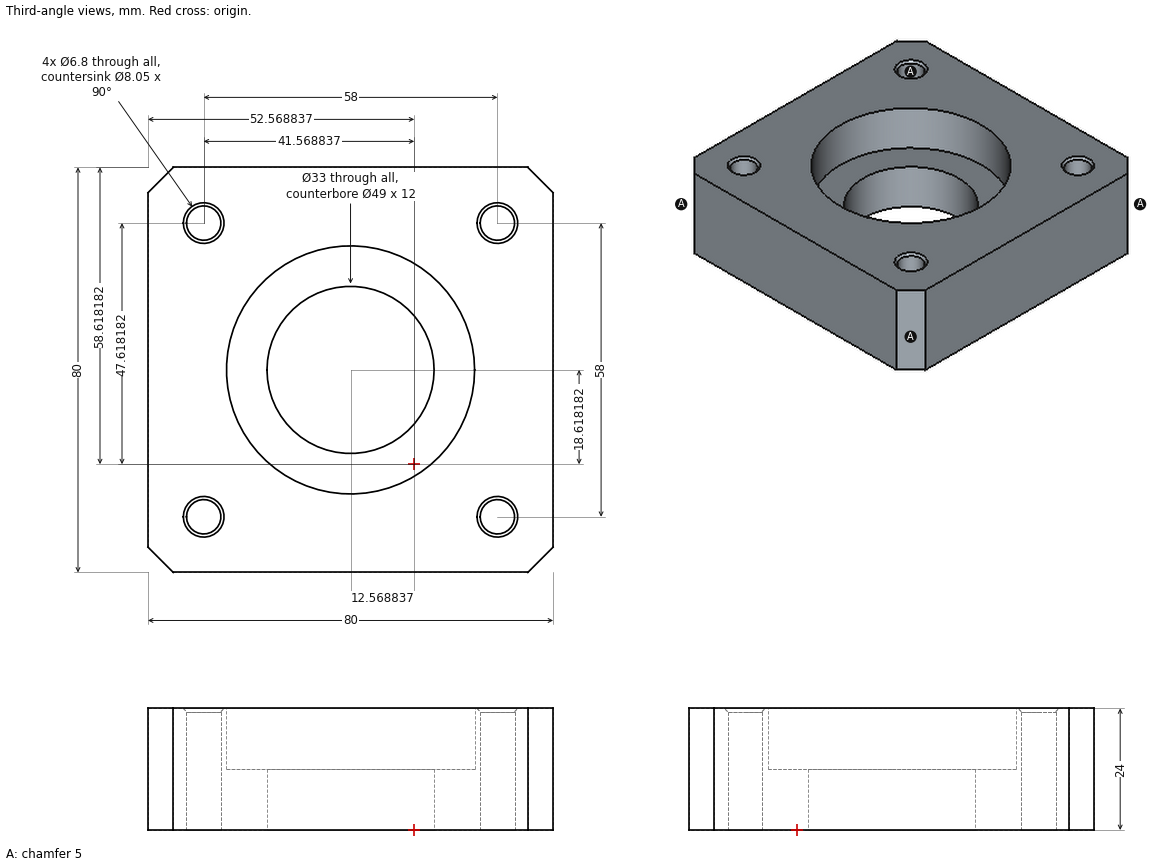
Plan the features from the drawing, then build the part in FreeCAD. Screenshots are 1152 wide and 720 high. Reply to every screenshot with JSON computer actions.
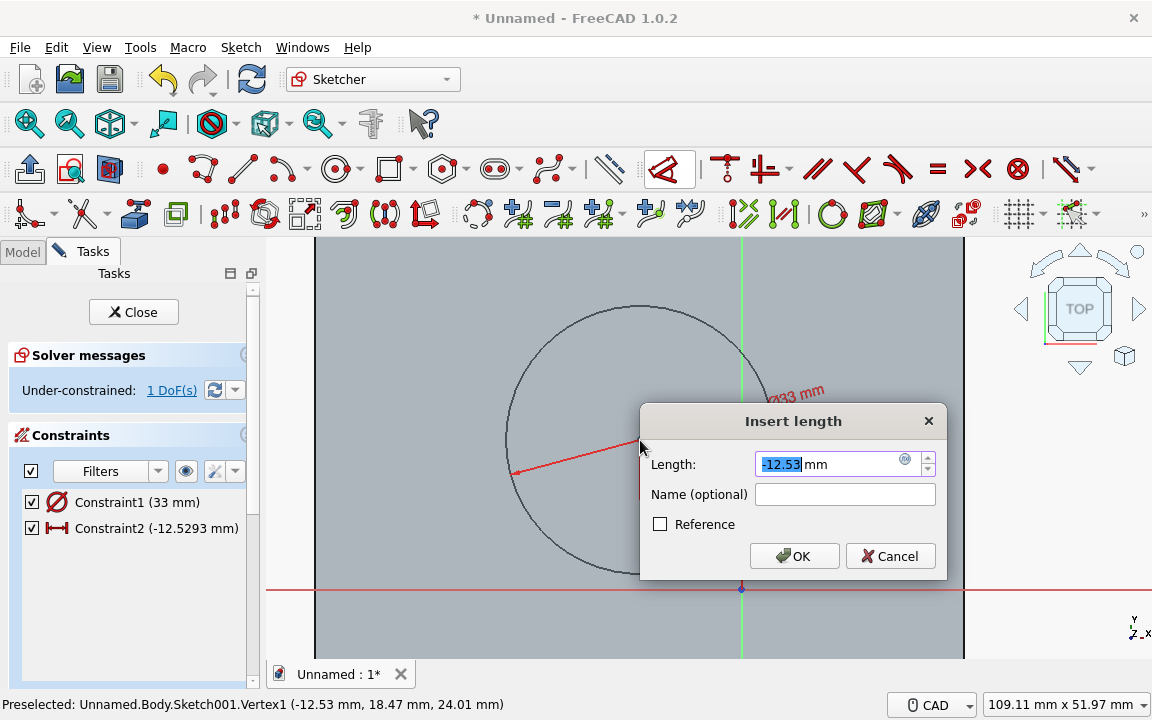
{"action": "type", "text": "-12.568837"}
{"action": "key", "text": "Return"}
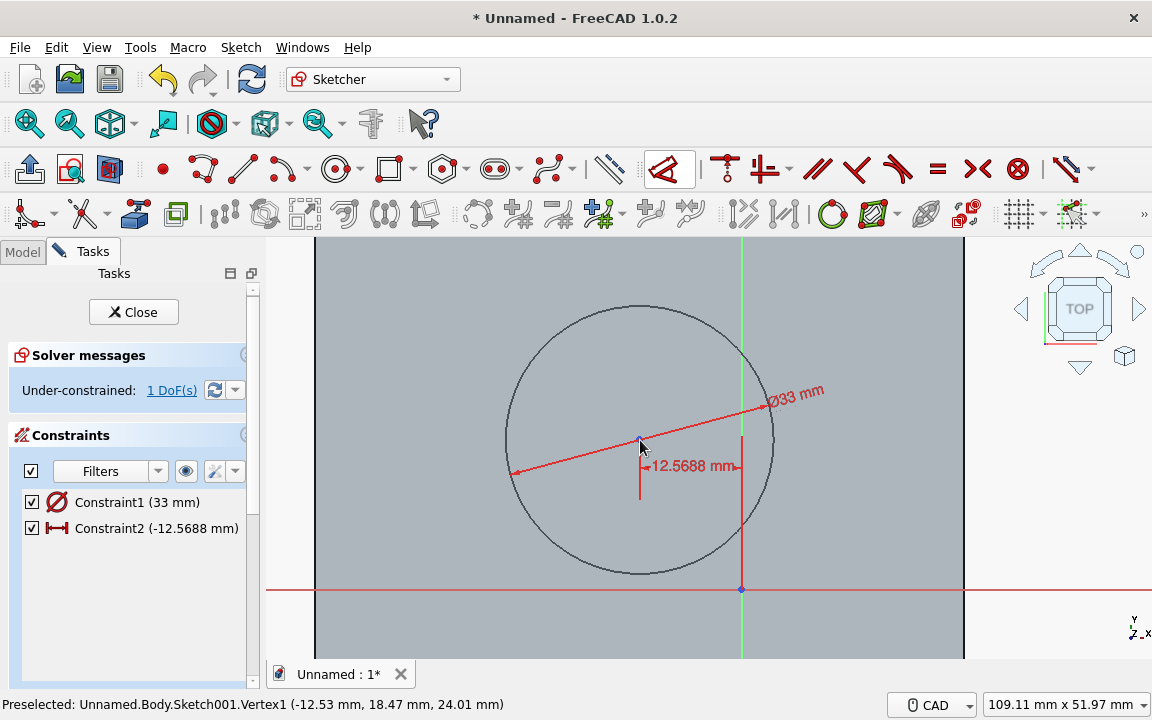
{"action": "left_click", "coordinate": [640, 440]}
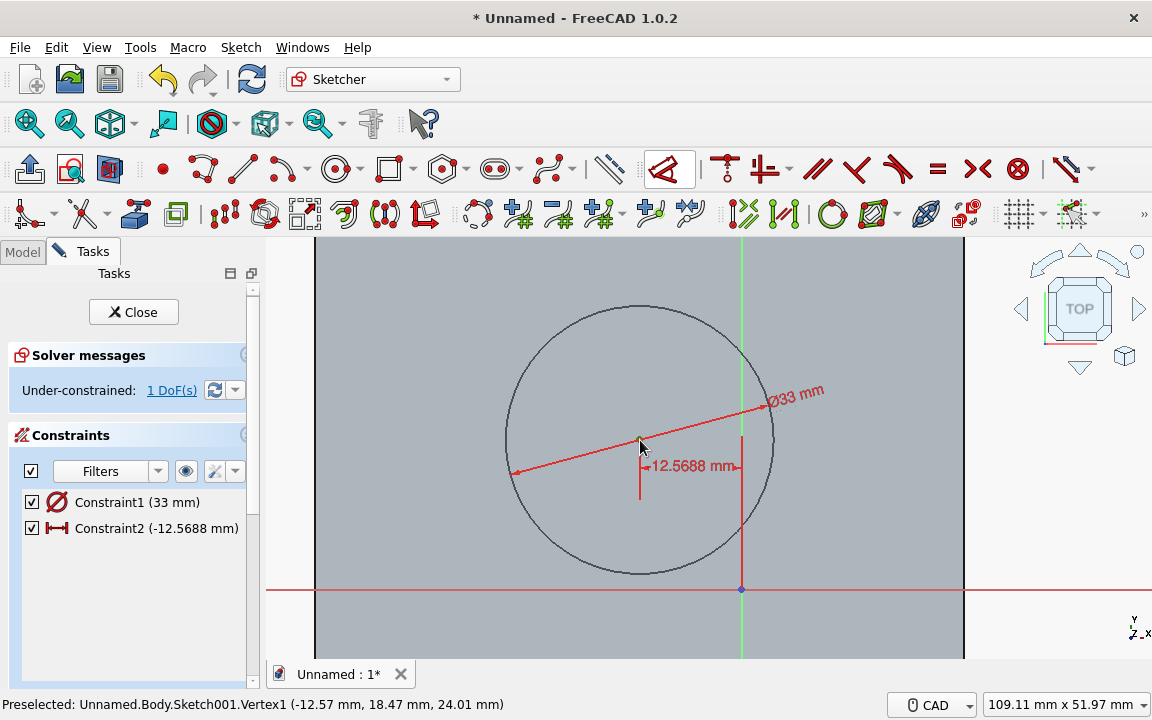
{"action": "key", "text": "i"}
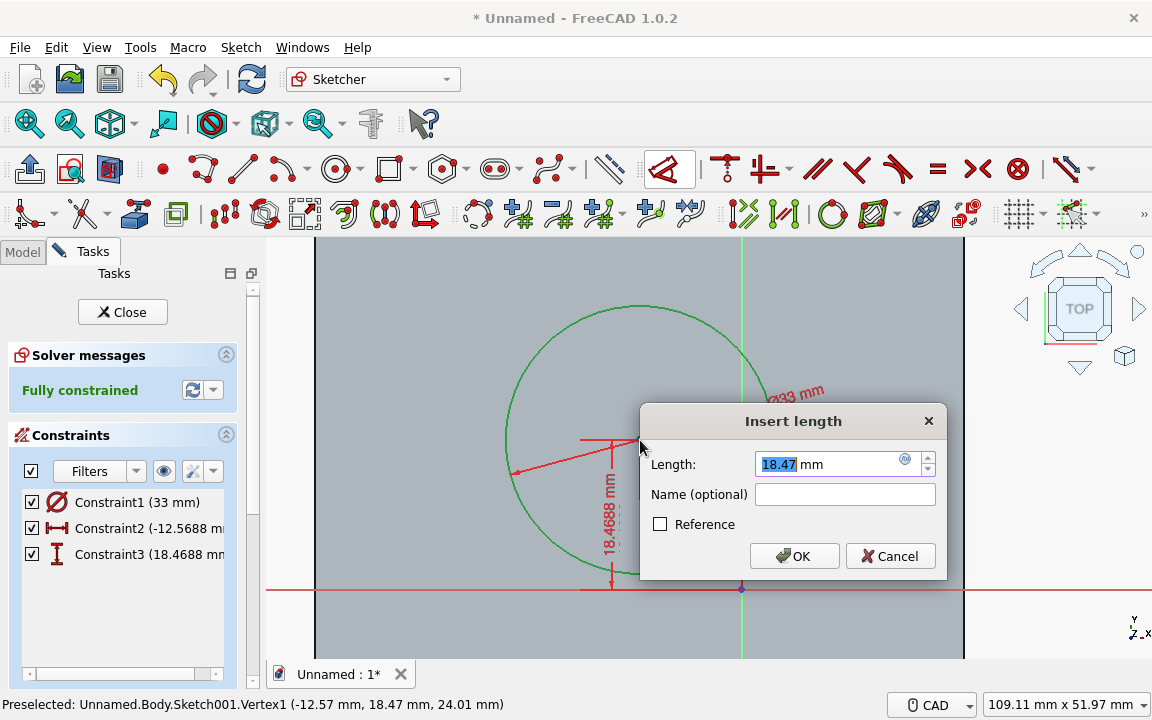
{"action": "type", "text": "18.618182"}
{"action": "key", "text": "Return"}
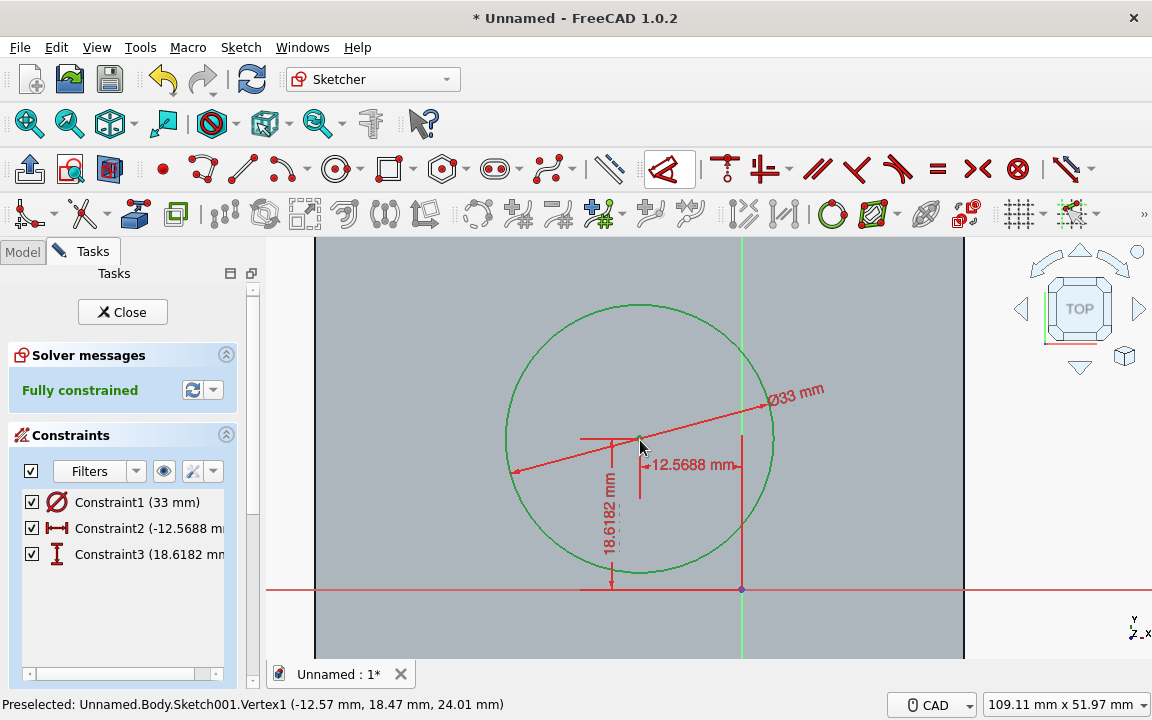
{"action": "left_click", "coordinate": [123, 312]}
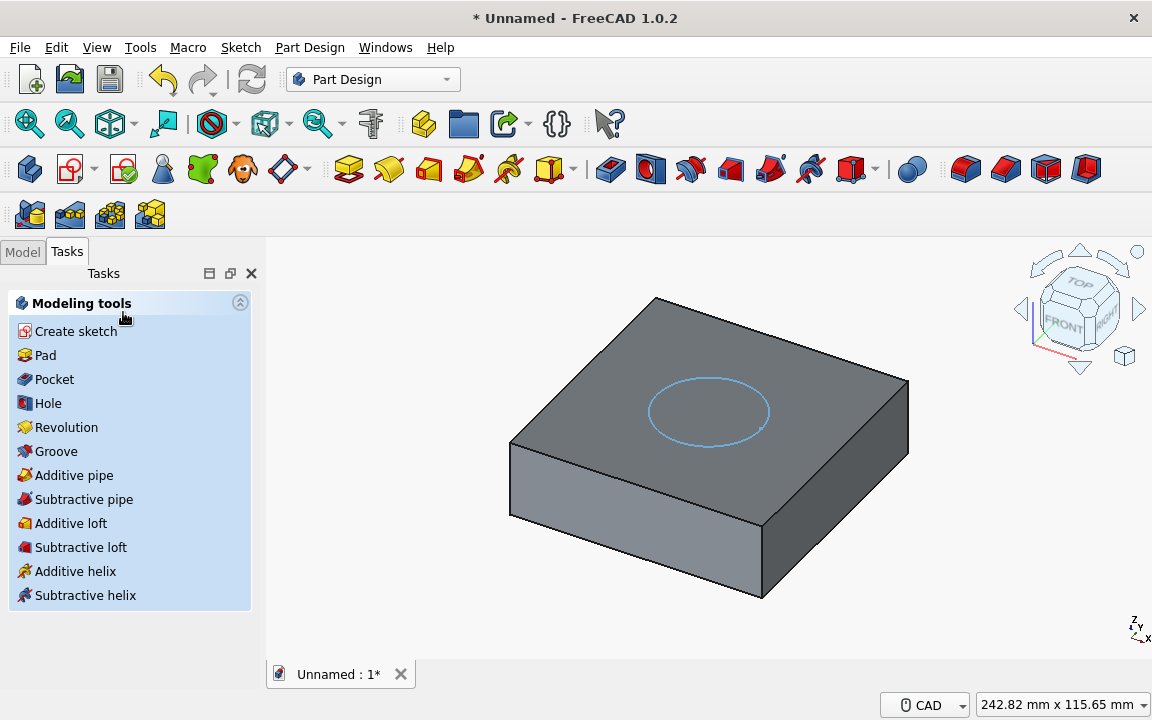
{"action": "left_click", "coordinate": [652, 170]}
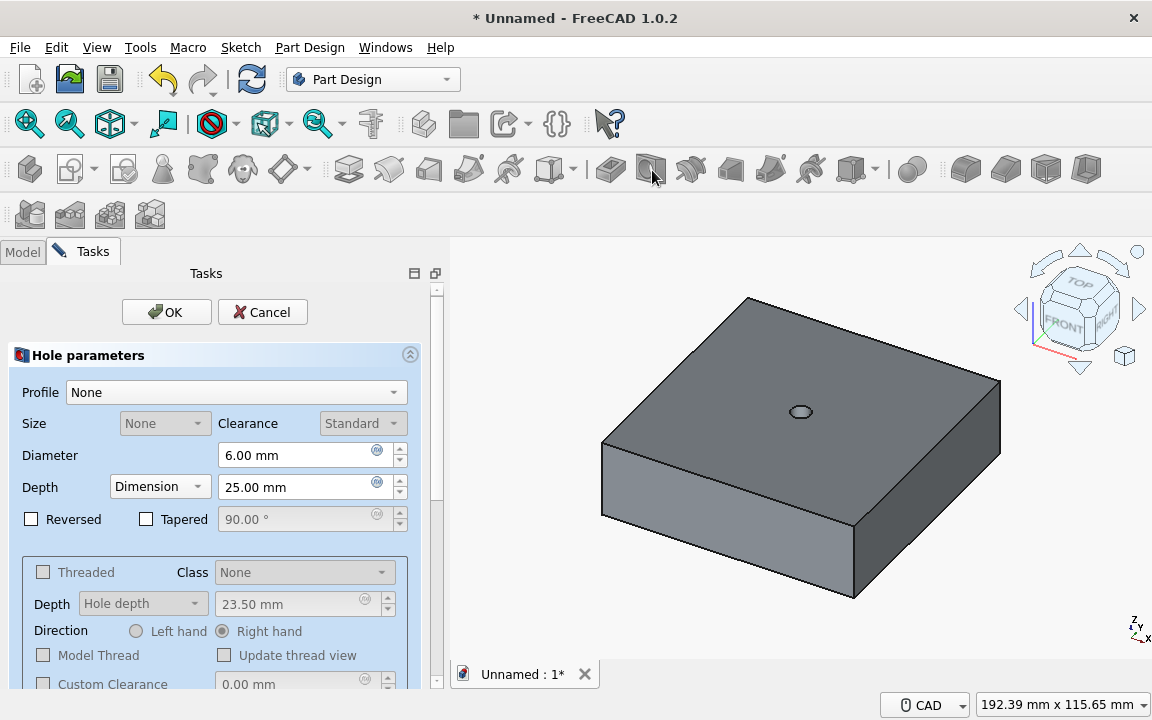
{"action": "triple_click", "coordinate": [305, 455]}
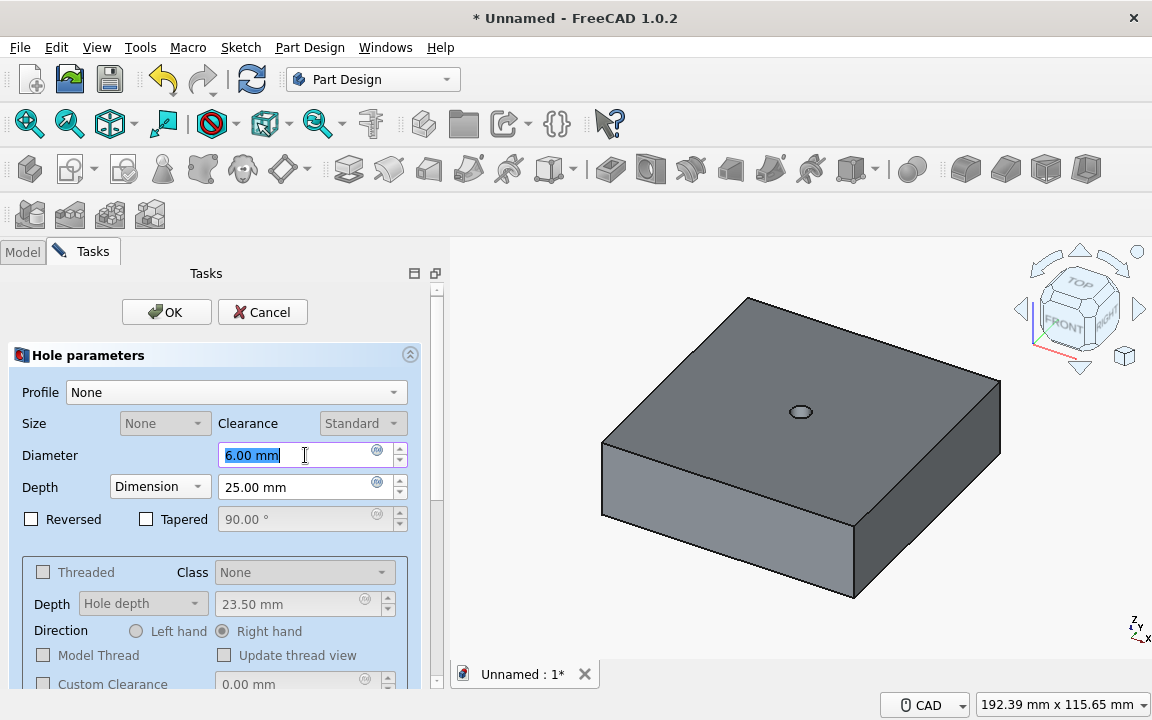
{"action": "type", "text": "33"}
{"action": "key", "text": "Tab"}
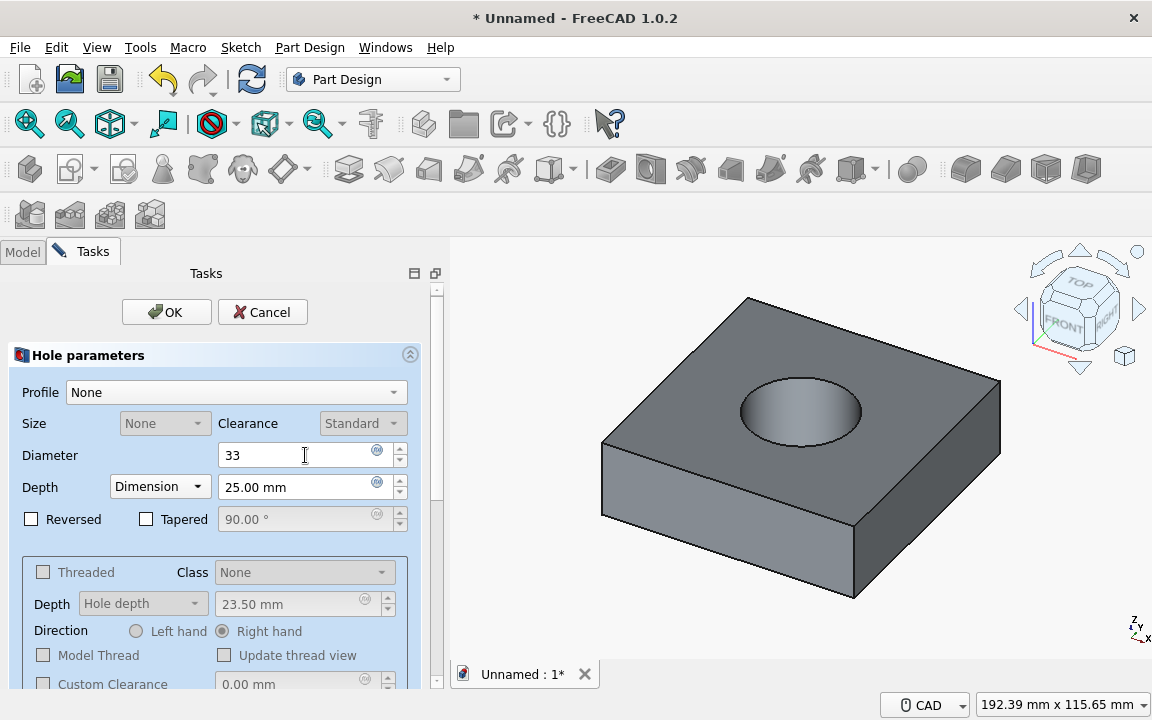
{"action": "left_click", "coordinate": [161, 486]}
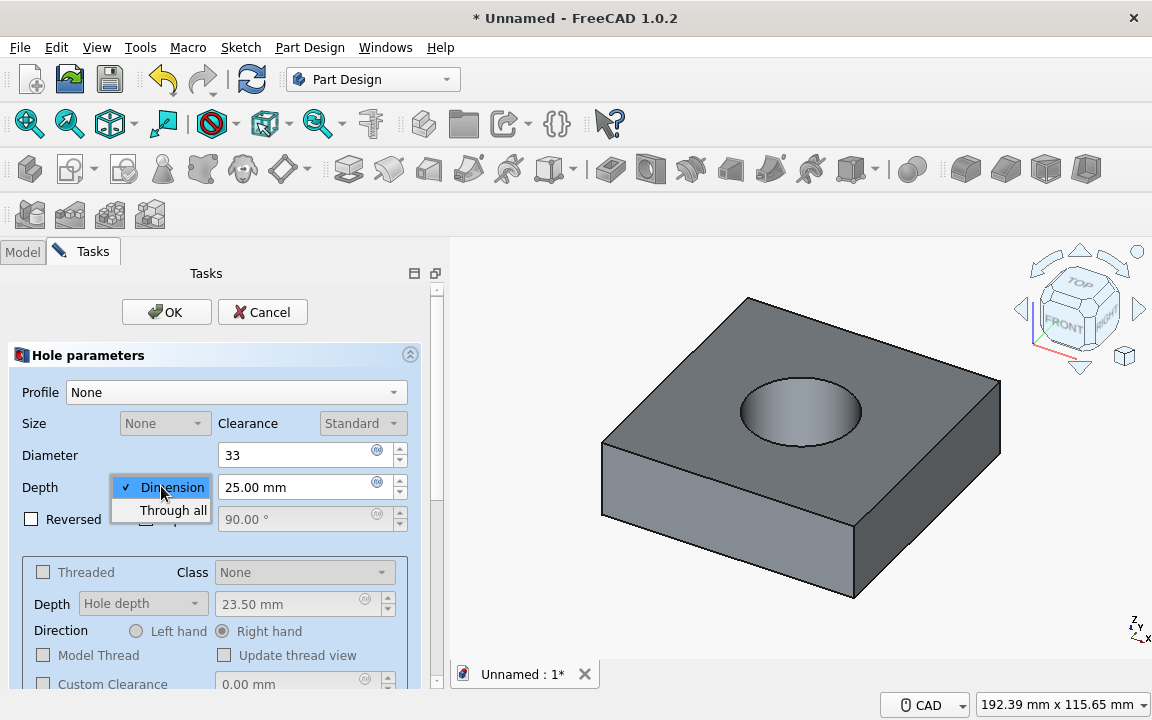
{"action": "left_click", "coordinate": [160, 510]}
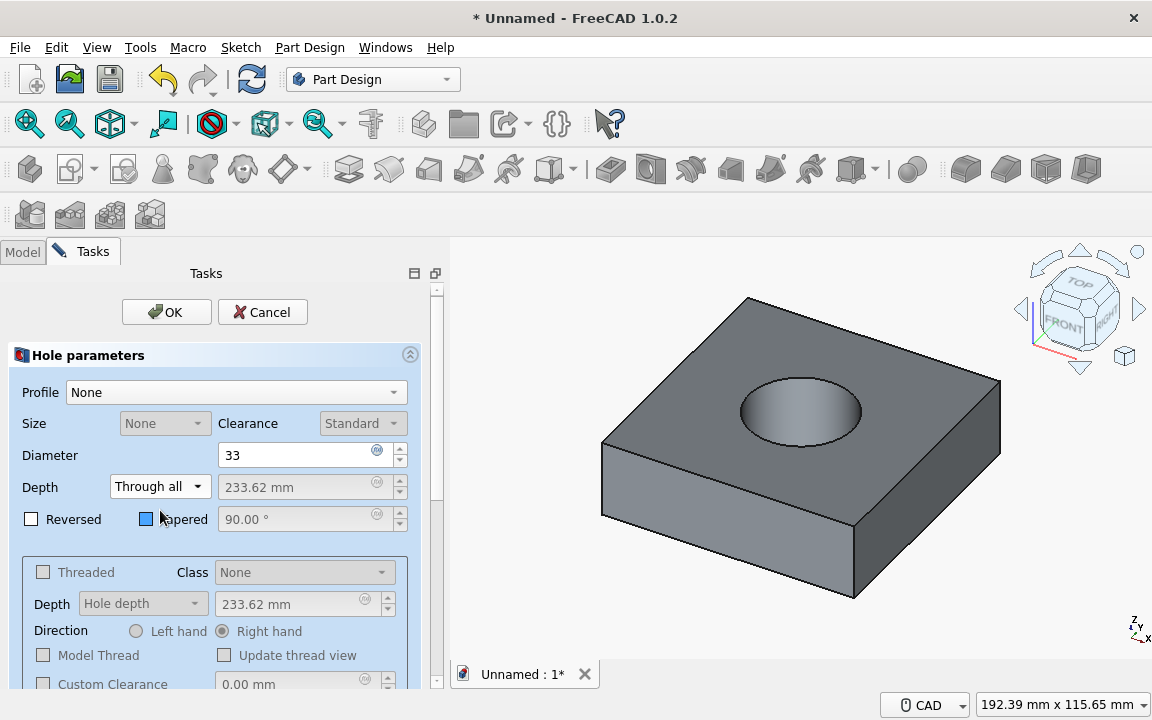
{"action": "scroll", "coordinate": [437, 486], "scroll_direction": "down", "scroll_amount": 3}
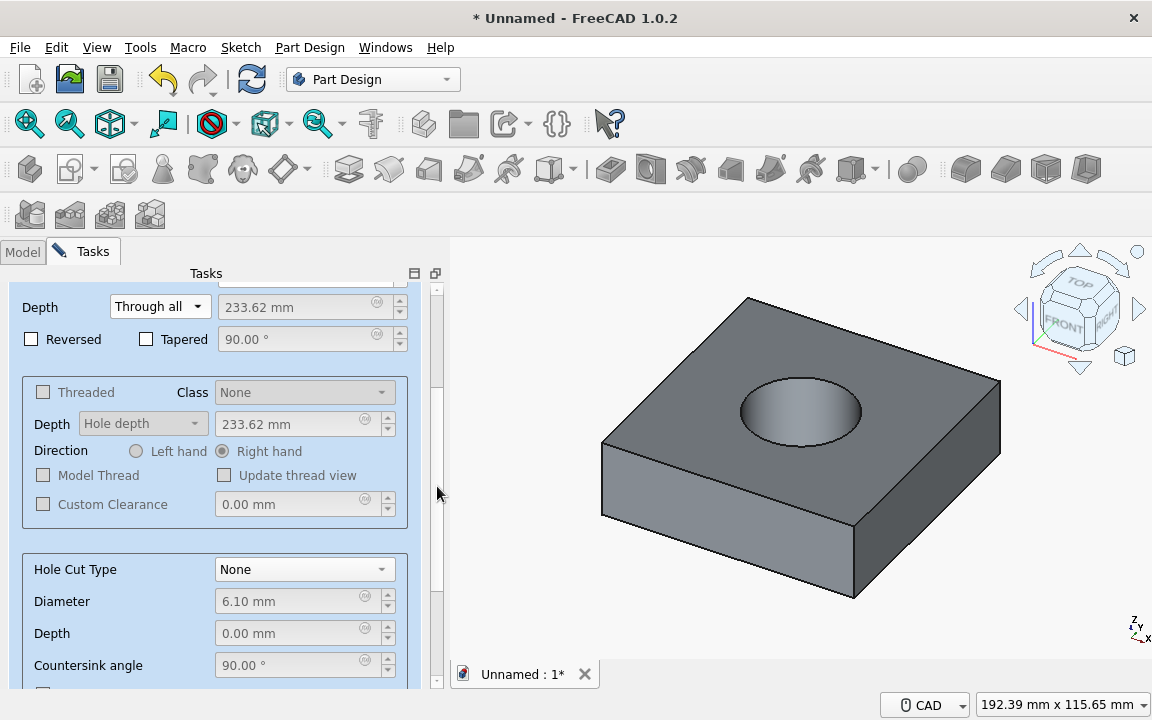
{"action": "left_click", "coordinate": [306, 570]}